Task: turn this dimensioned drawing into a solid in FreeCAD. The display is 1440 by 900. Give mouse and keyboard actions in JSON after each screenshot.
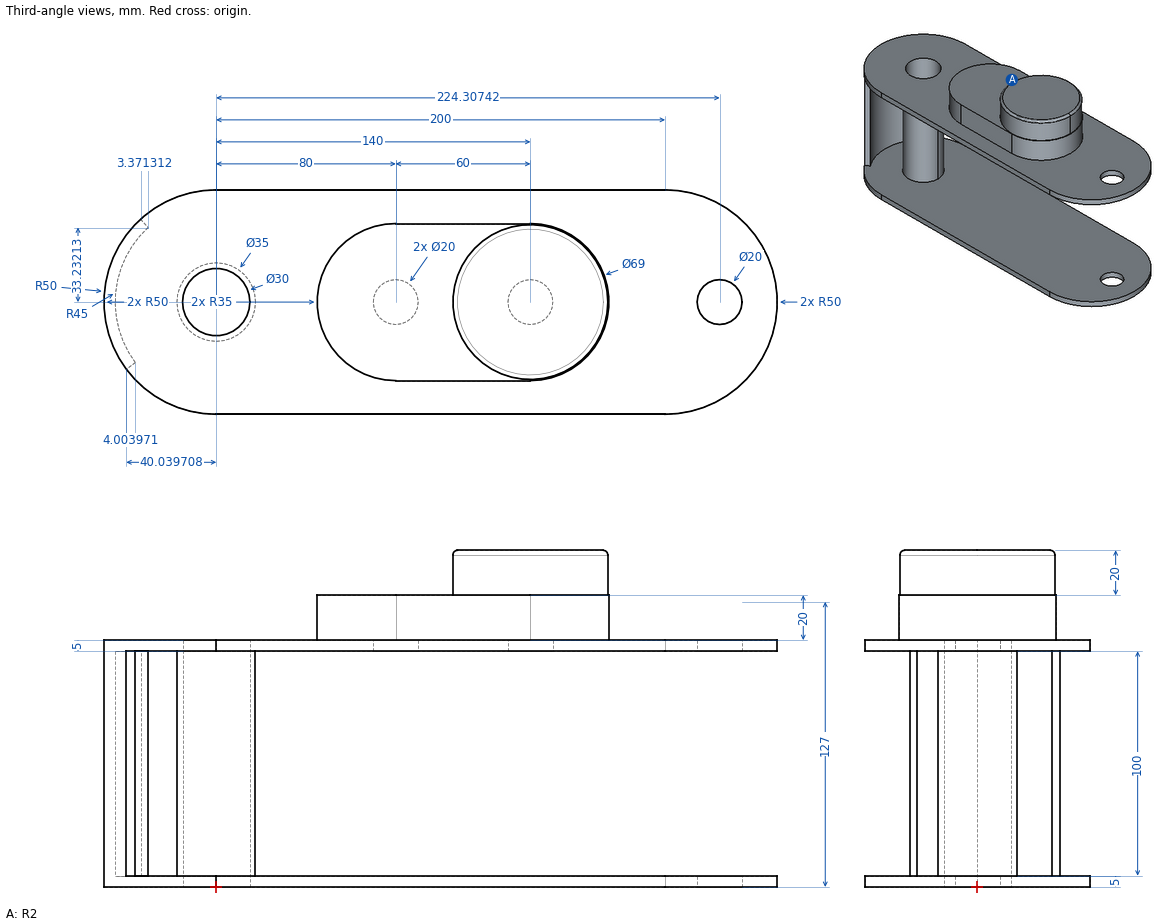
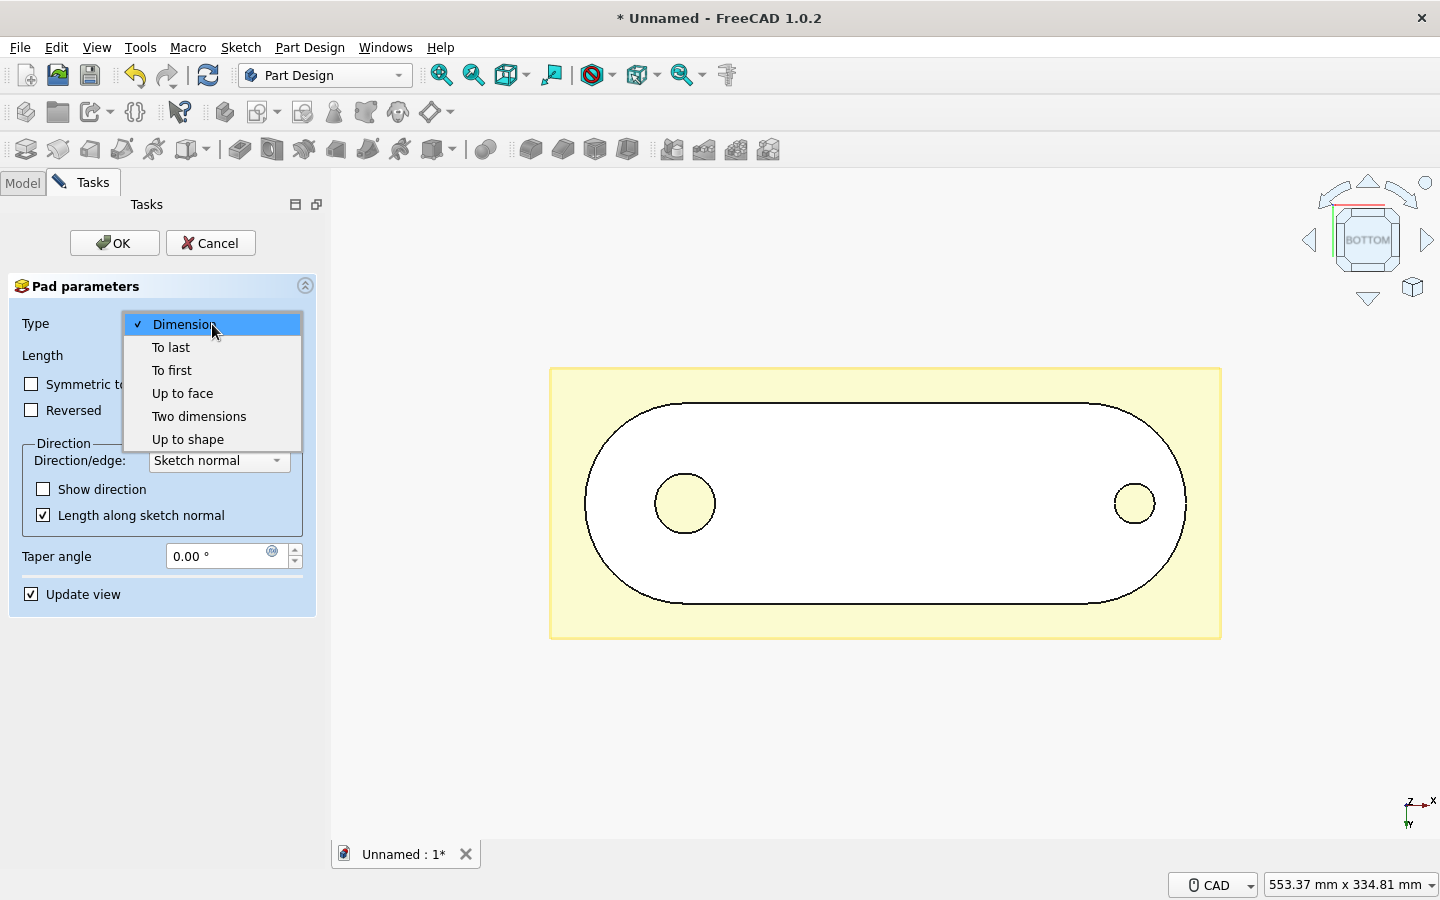
{"action": "left_click", "coordinate": [212, 370]}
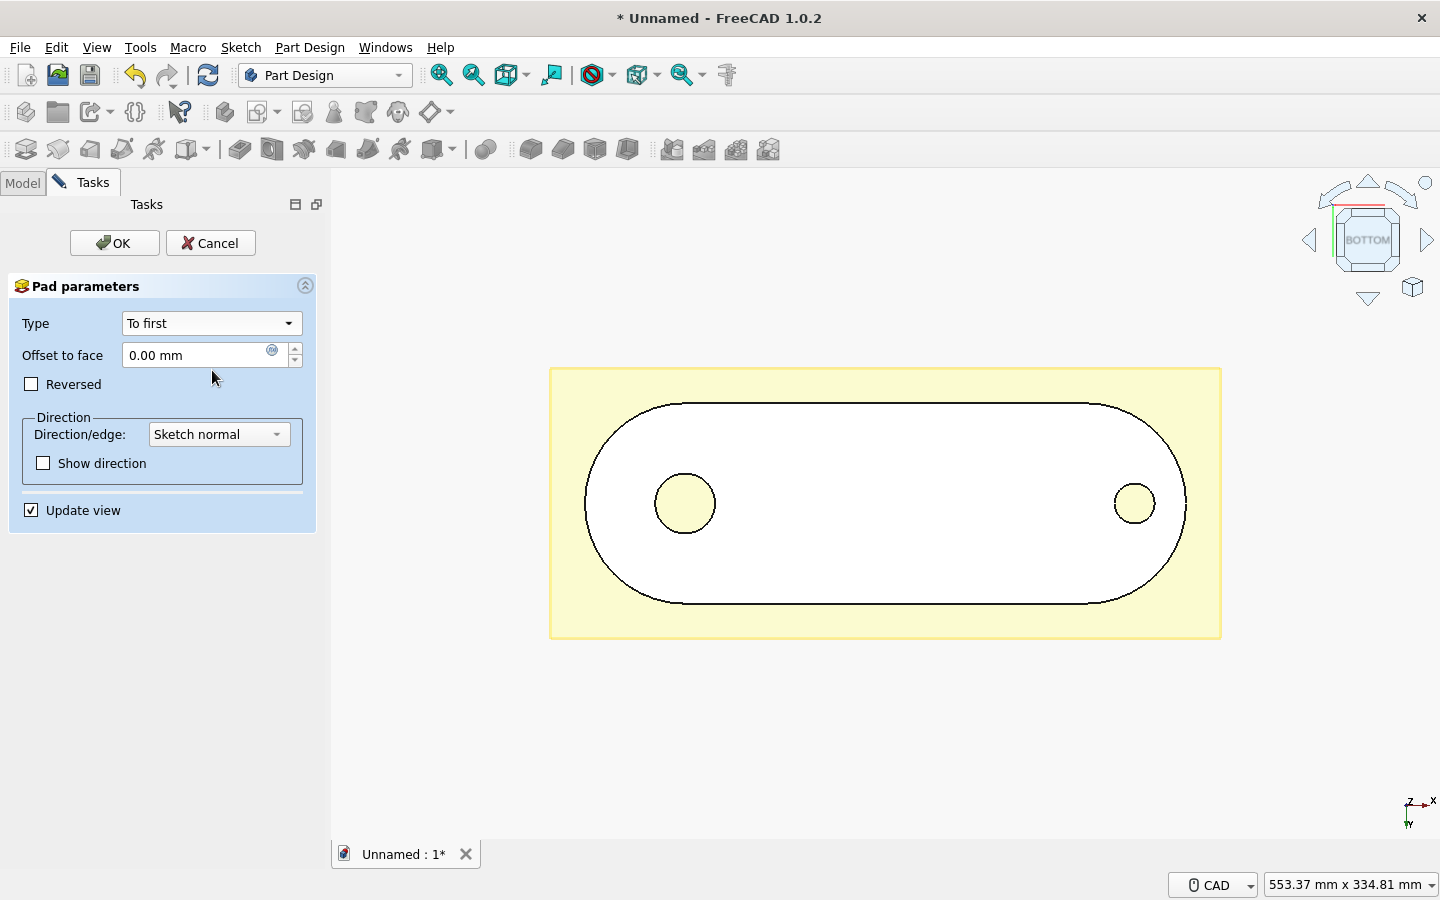
{"action": "left_click", "coordinate": [115, 243]}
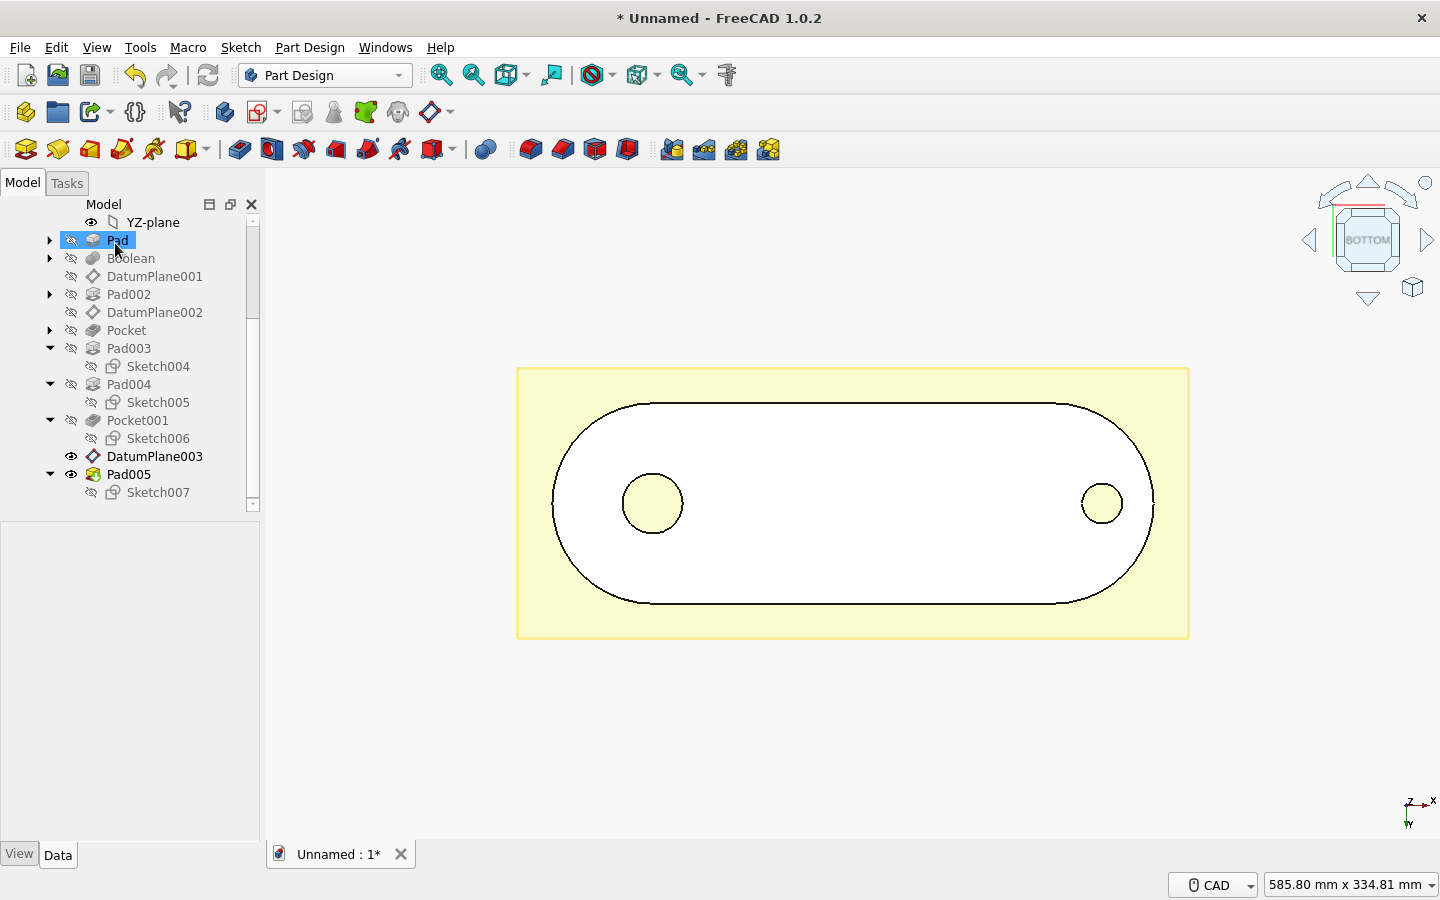
{"action": "left_click", "coordinate": [116, 456]}
{"action": "key", "text": "space"}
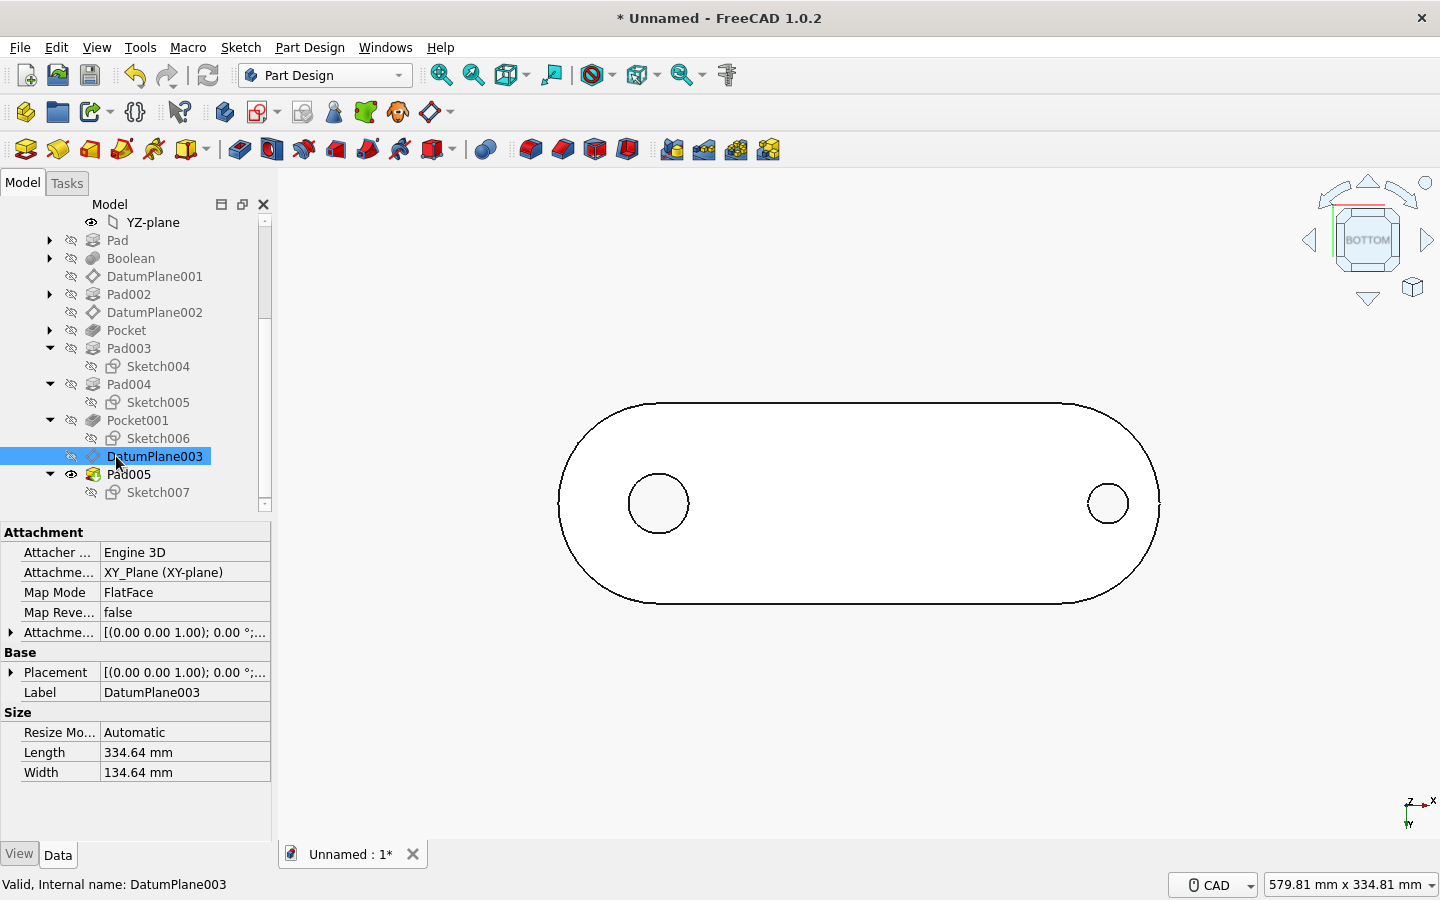
{"action": "key", "text": "0"}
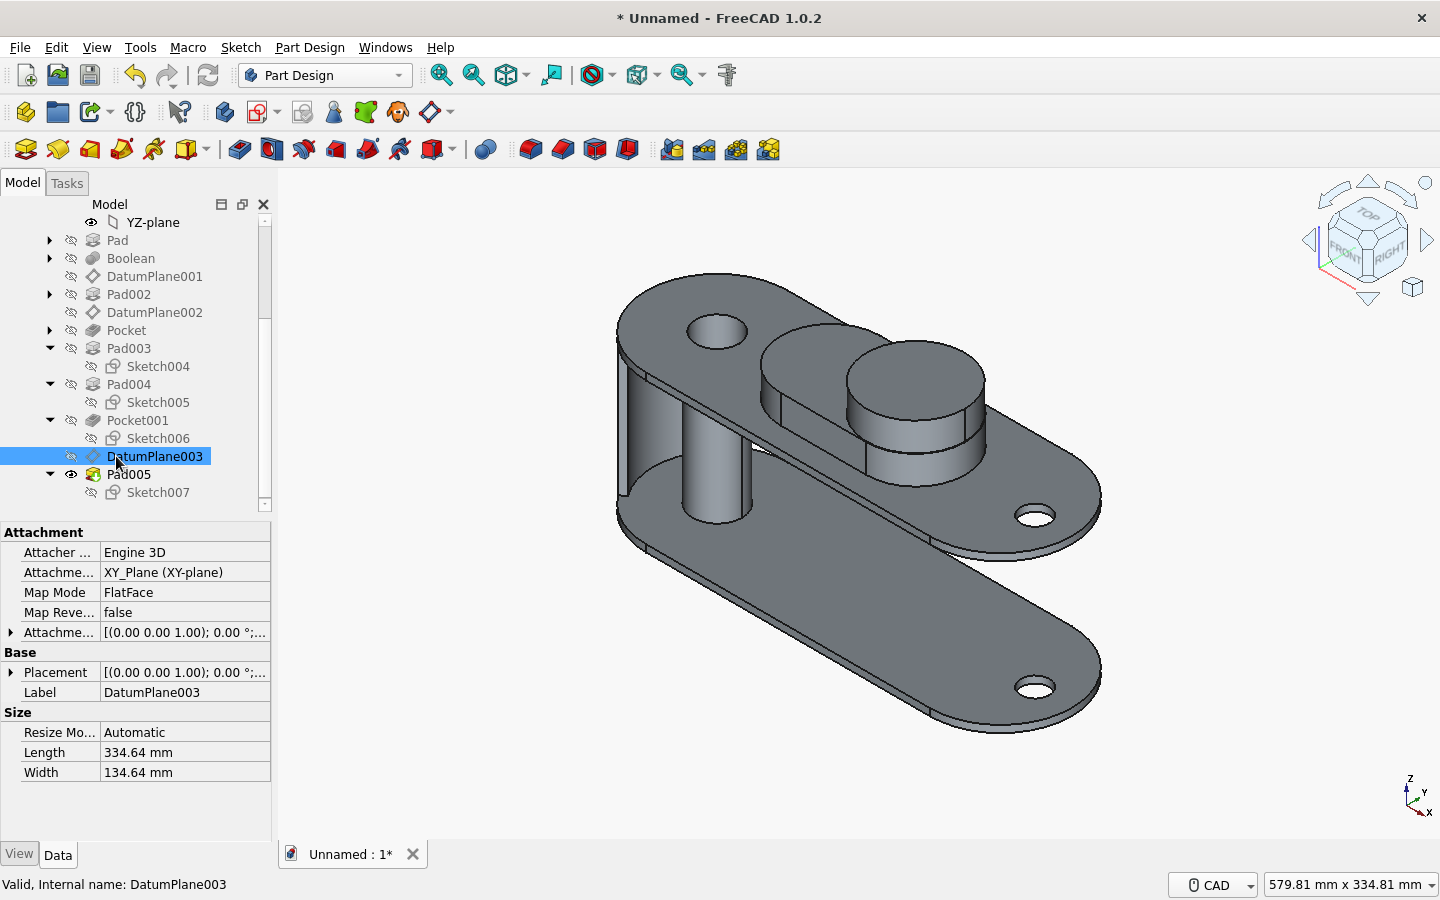
{"action": "left_click", "coordinate": [854, 398]}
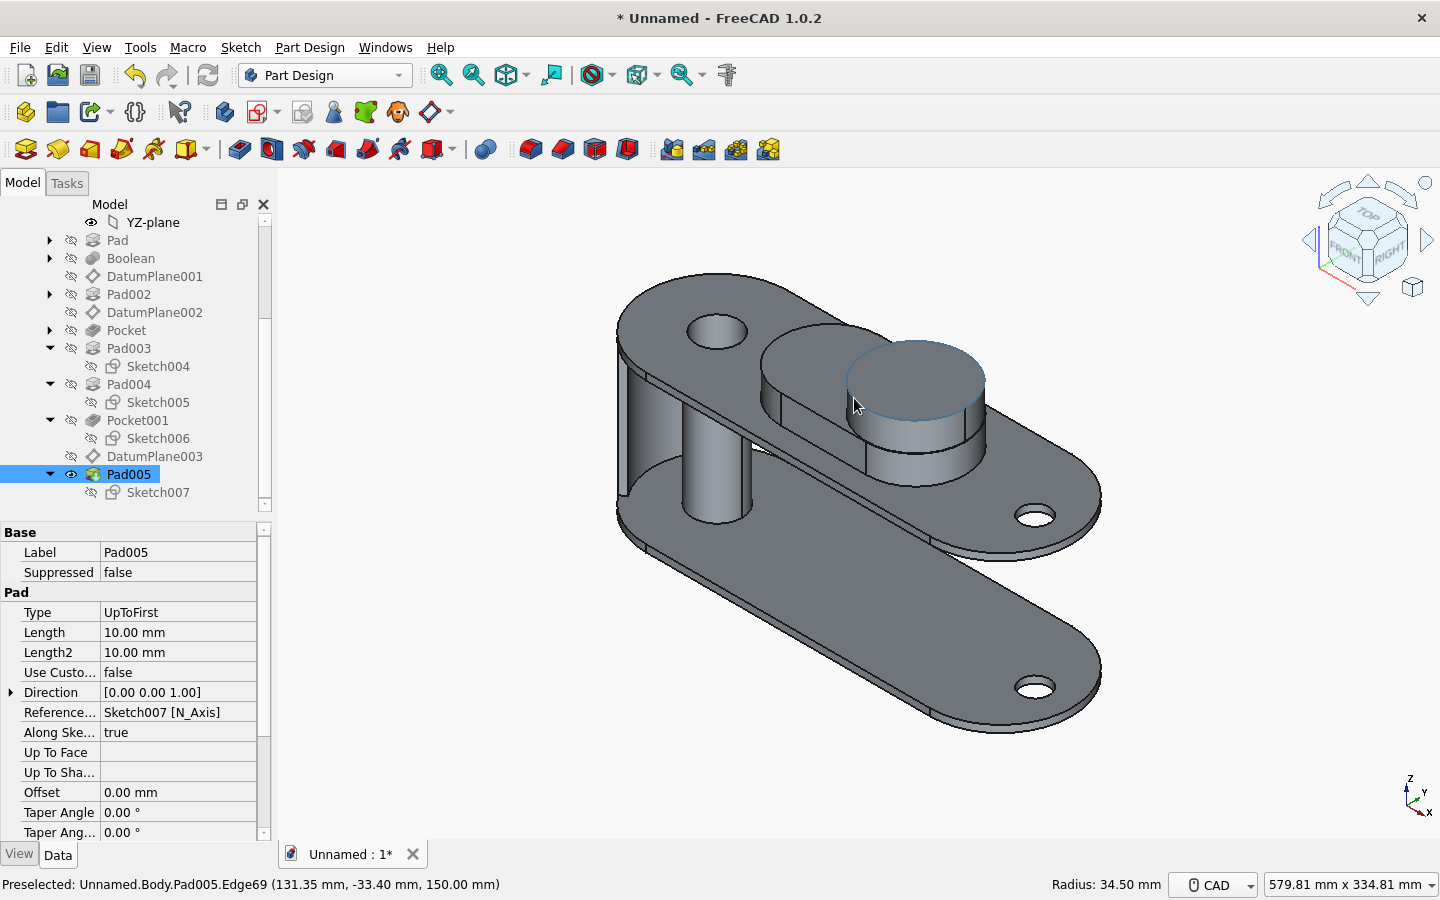
{"action": "left_click", "coordinate": [532, 150]}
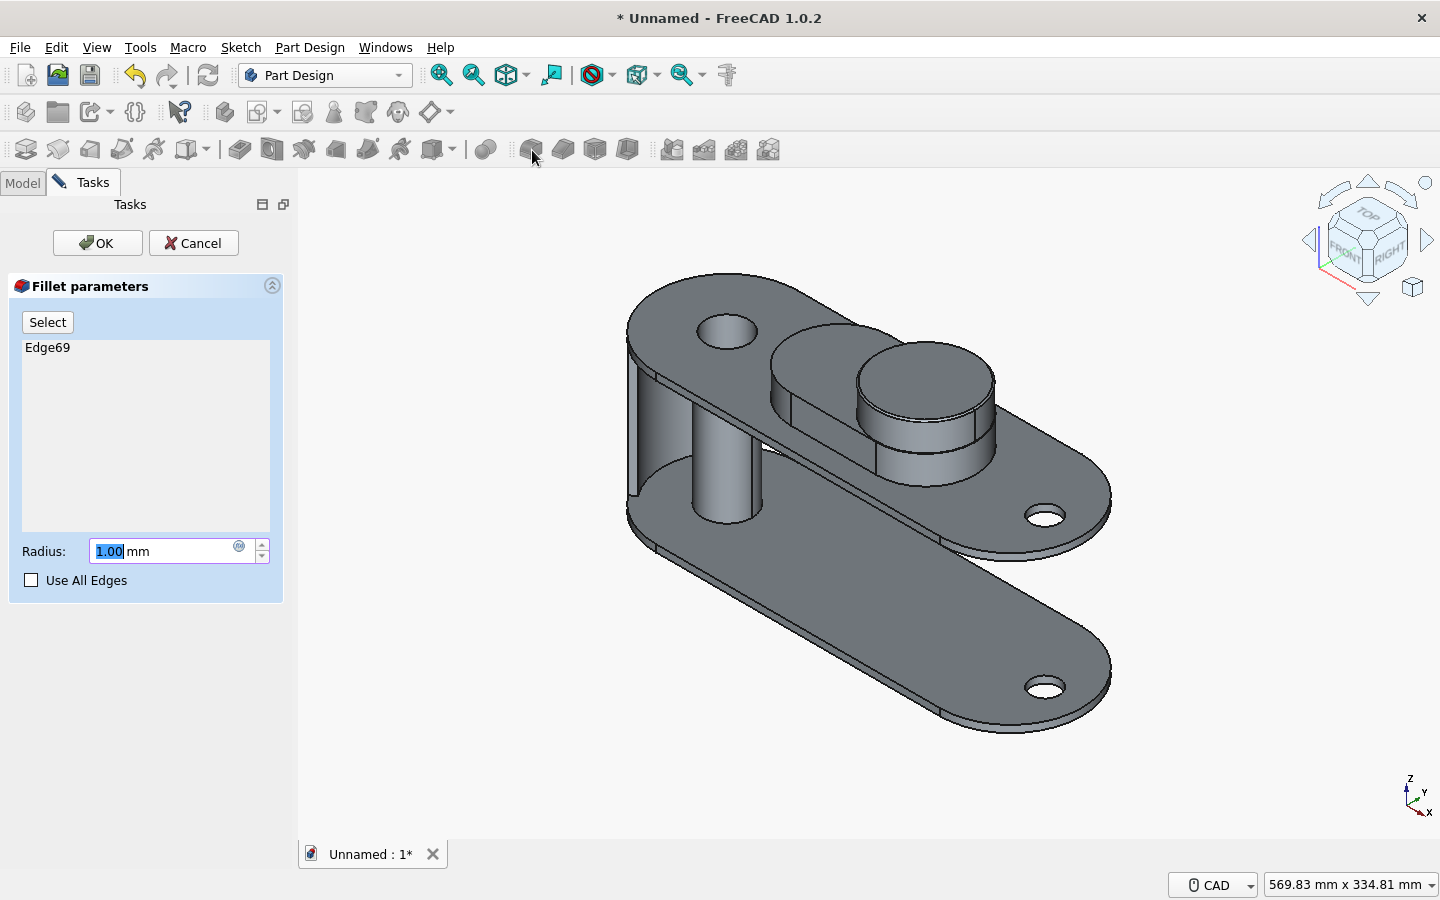
{"action": "type", "text": "2"}
{"action": "key", "text": "Tab"}